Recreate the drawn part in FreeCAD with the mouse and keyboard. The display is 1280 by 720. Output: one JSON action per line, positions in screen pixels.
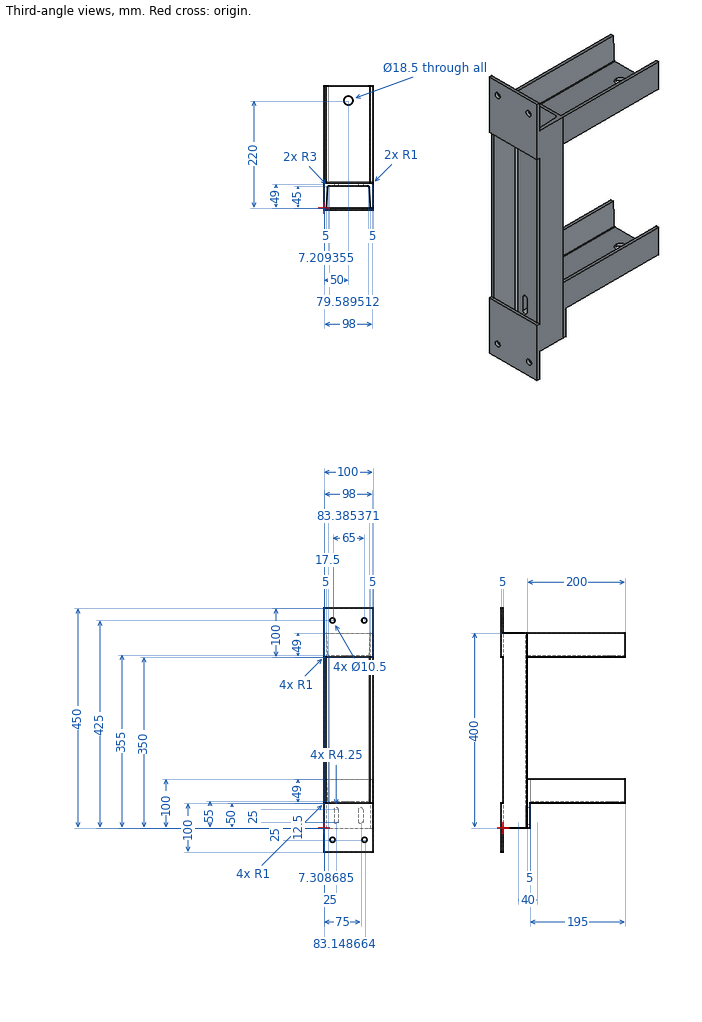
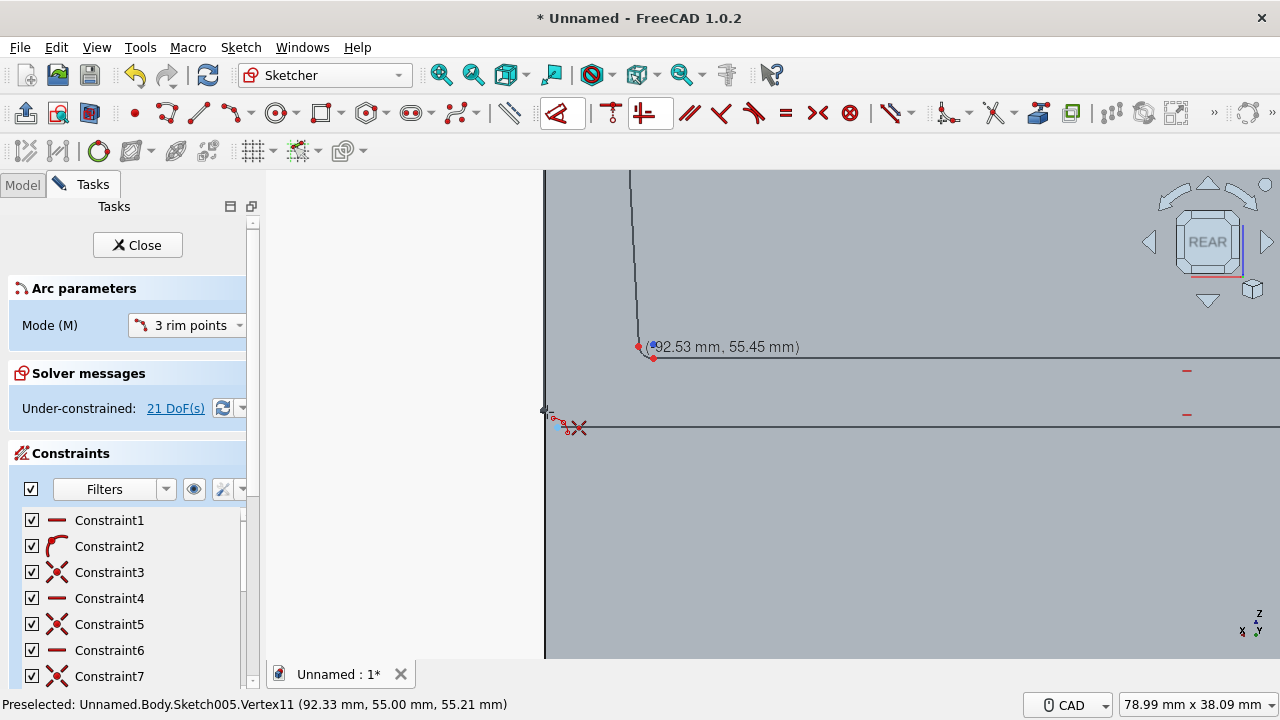
{"action": "left_click", "coordinate": [544, 410]}
{"action": "left_click", "coordinate": [558, 427]}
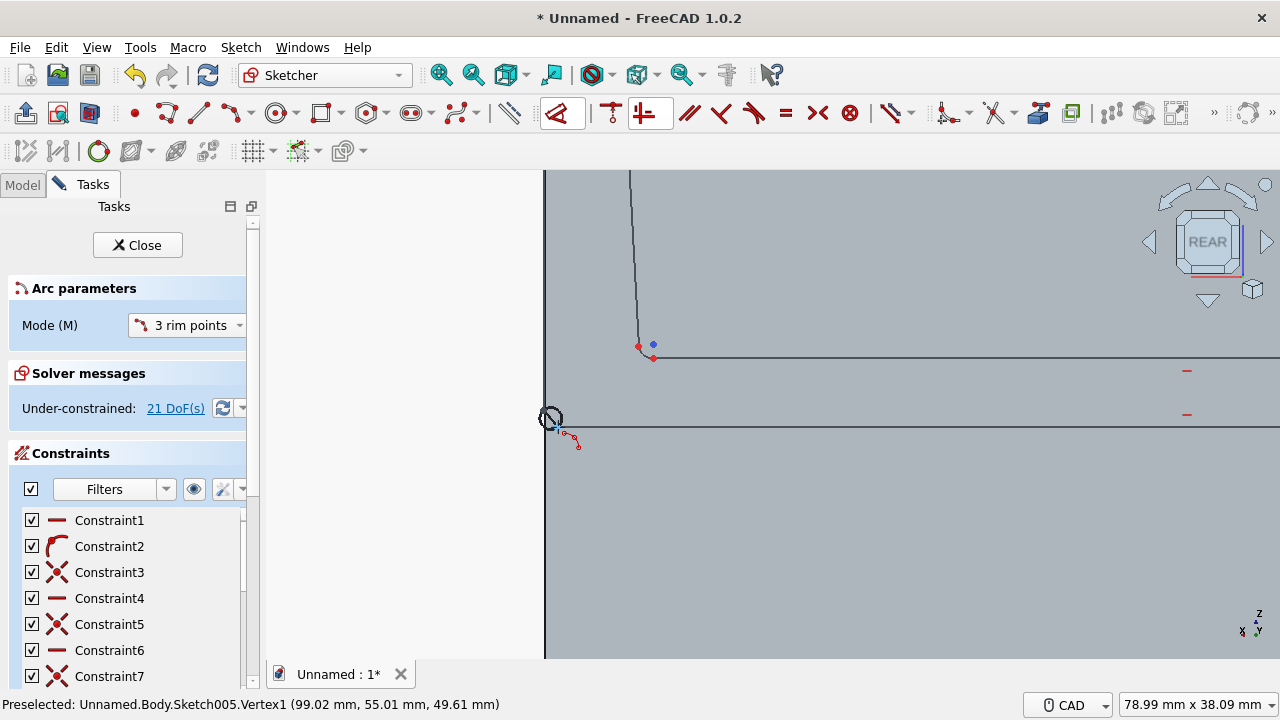
{"action": "scroll", "coordinate": [549, 418], "scroll_direction": "up", "scroll_amount": 8}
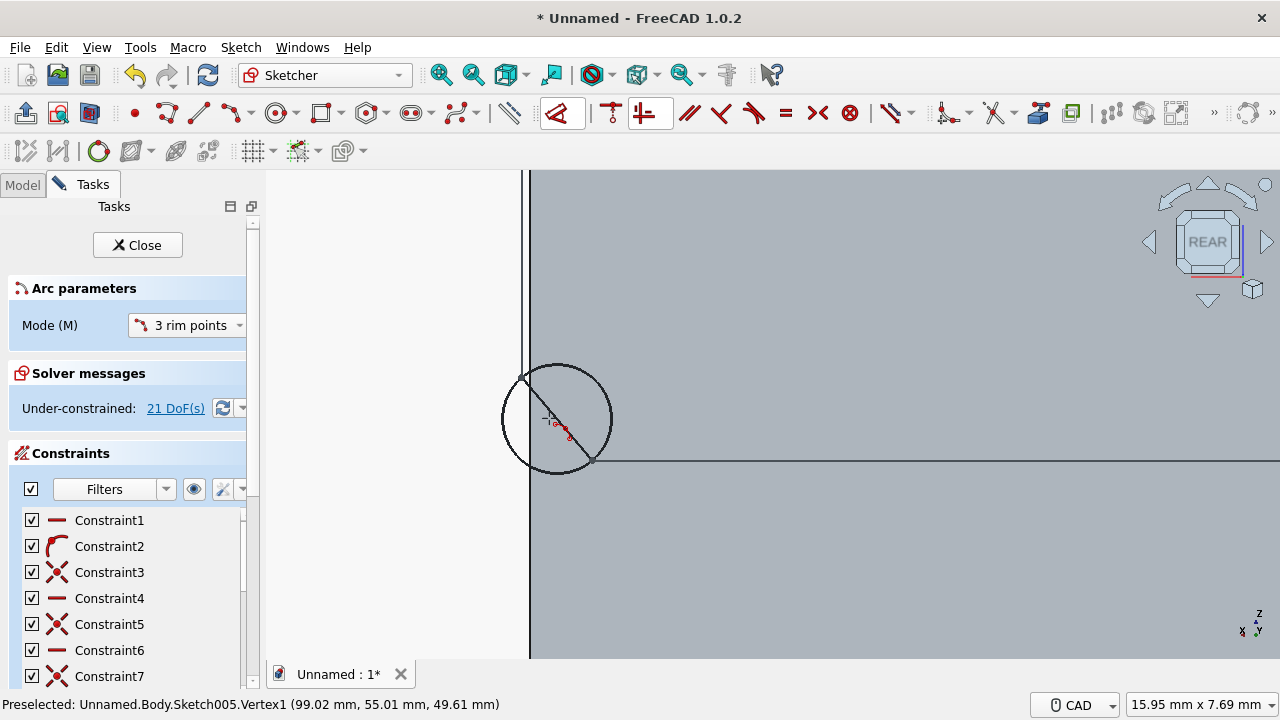
{"action": "left_click", "coordinate": [548, 417]}
{"action": "key", "text": "Escape"}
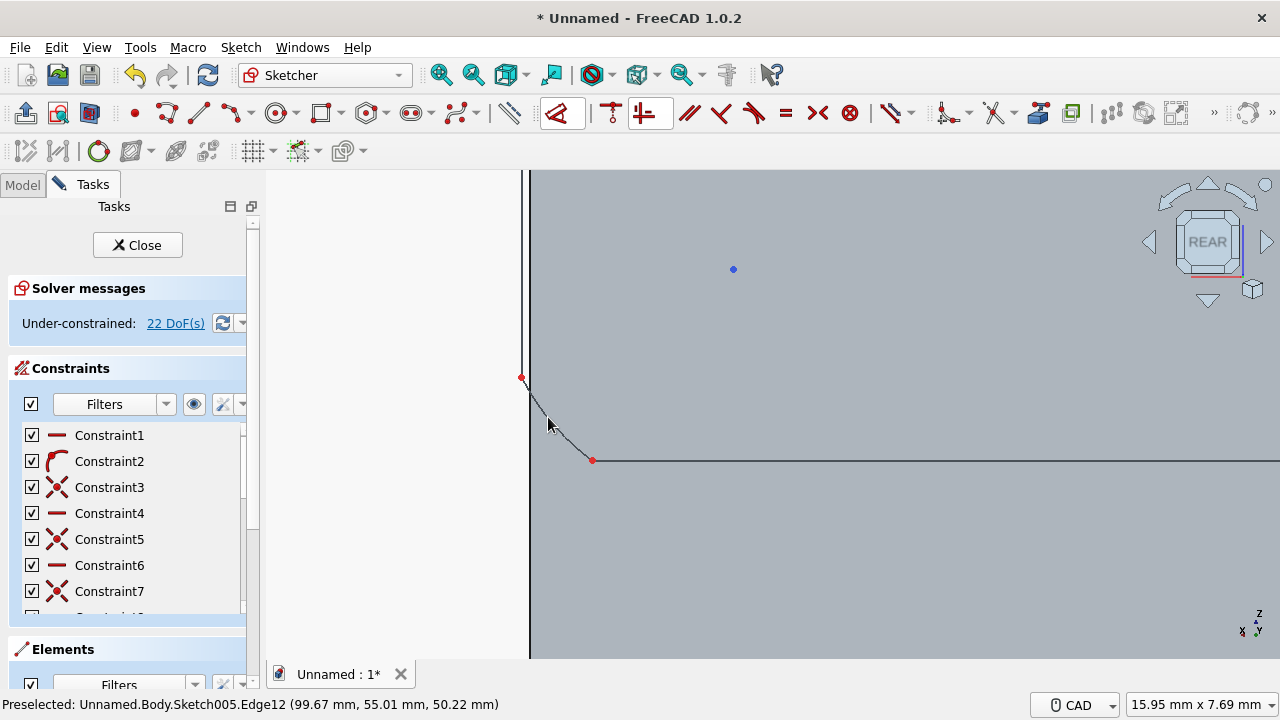
{"action": "scroll", "coordinate": [547, 413], "scroll_direction": "down", "scroll_amount": 15}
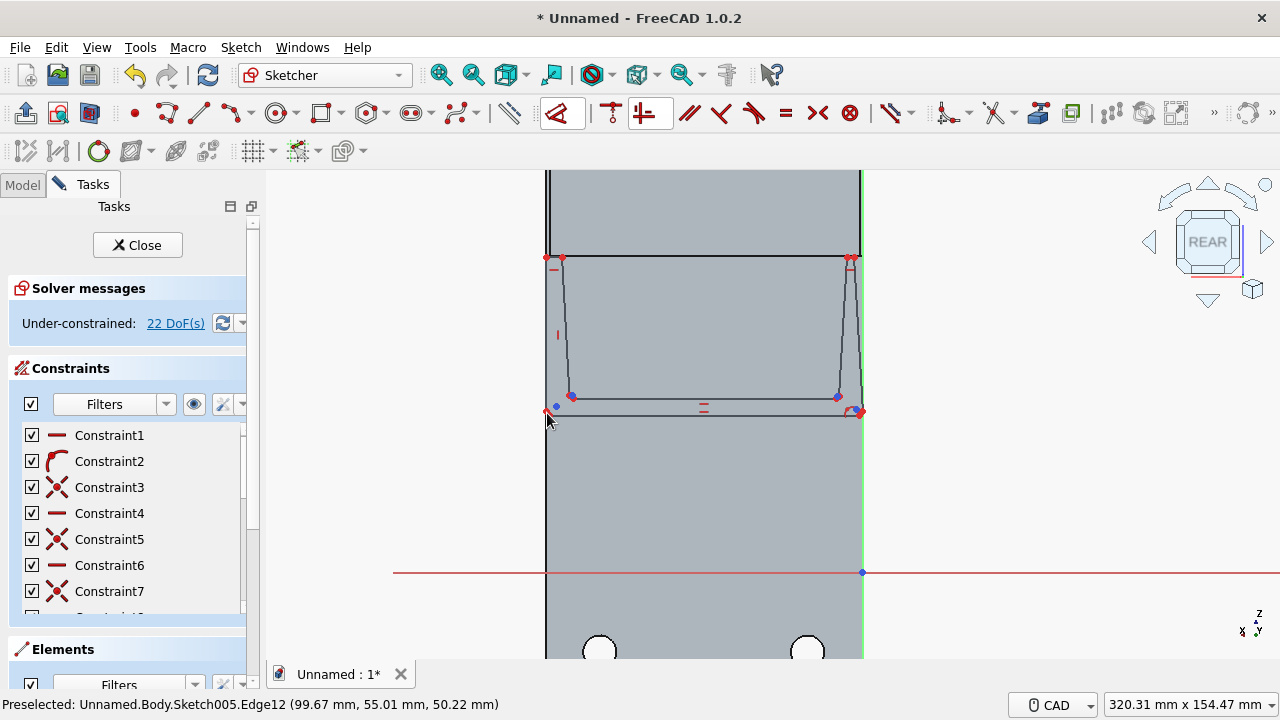
{"action": "left_click", "coordinate": [643, 416]}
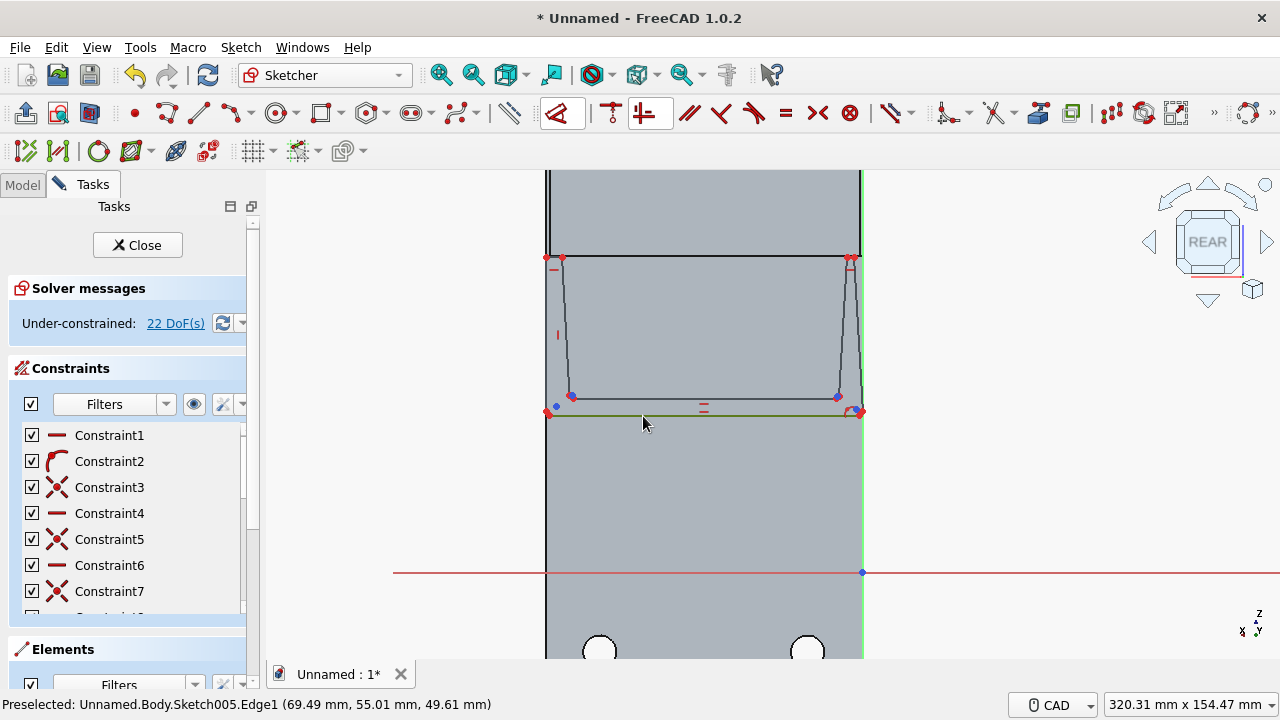
{"action": "scroll", "coordinate": [862, 414], "scroll_direction": "up", "scroll_amount": 9}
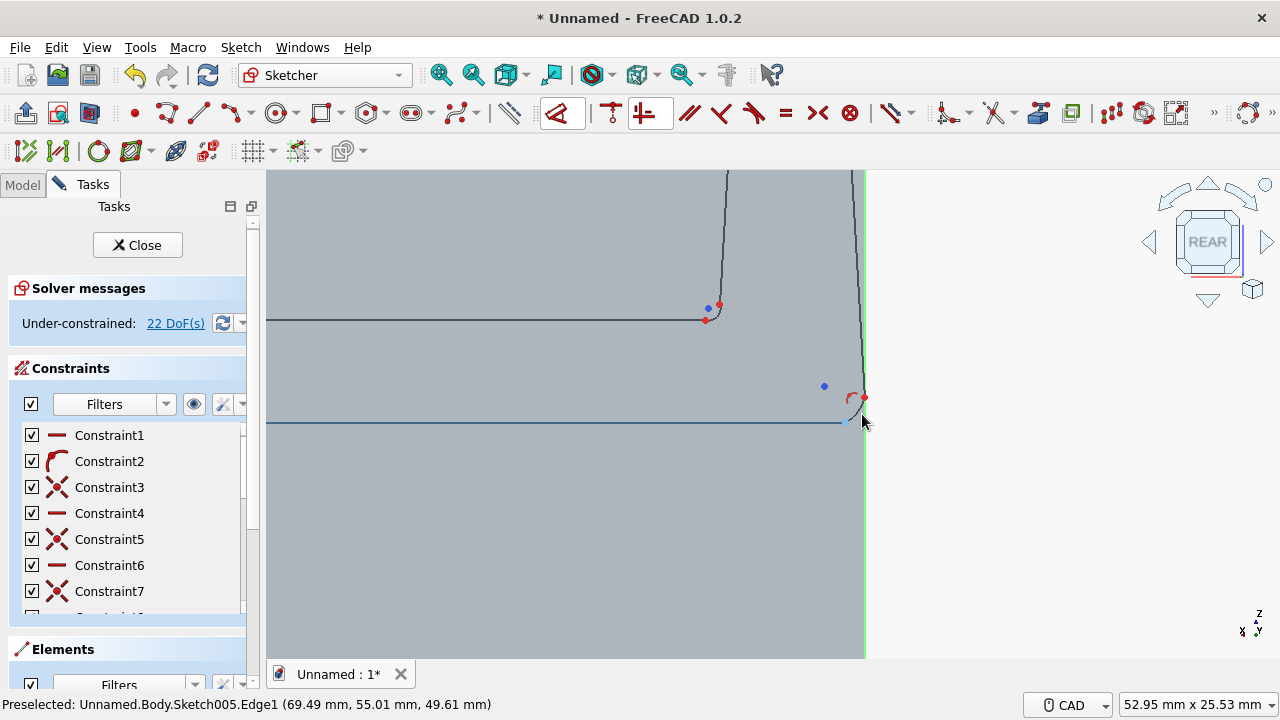
{"action": "left_click", "coordinate": [858, 412]}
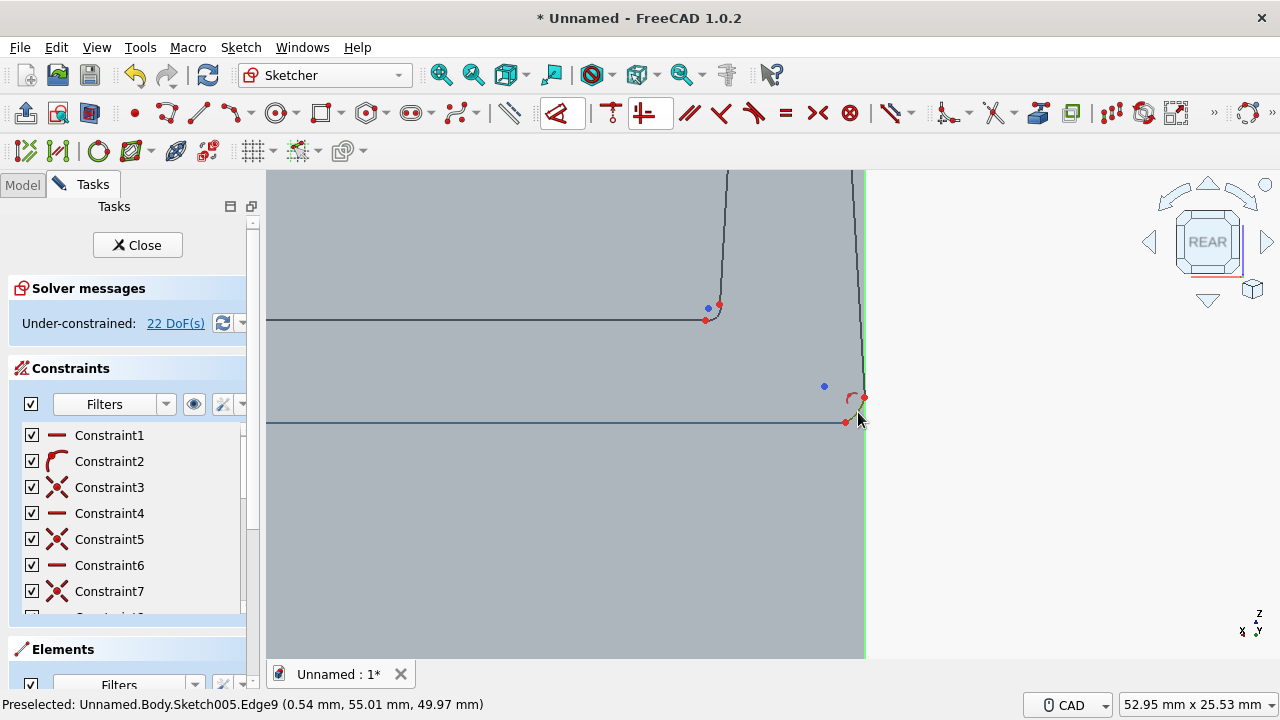
{"action": "key", "text": "t"}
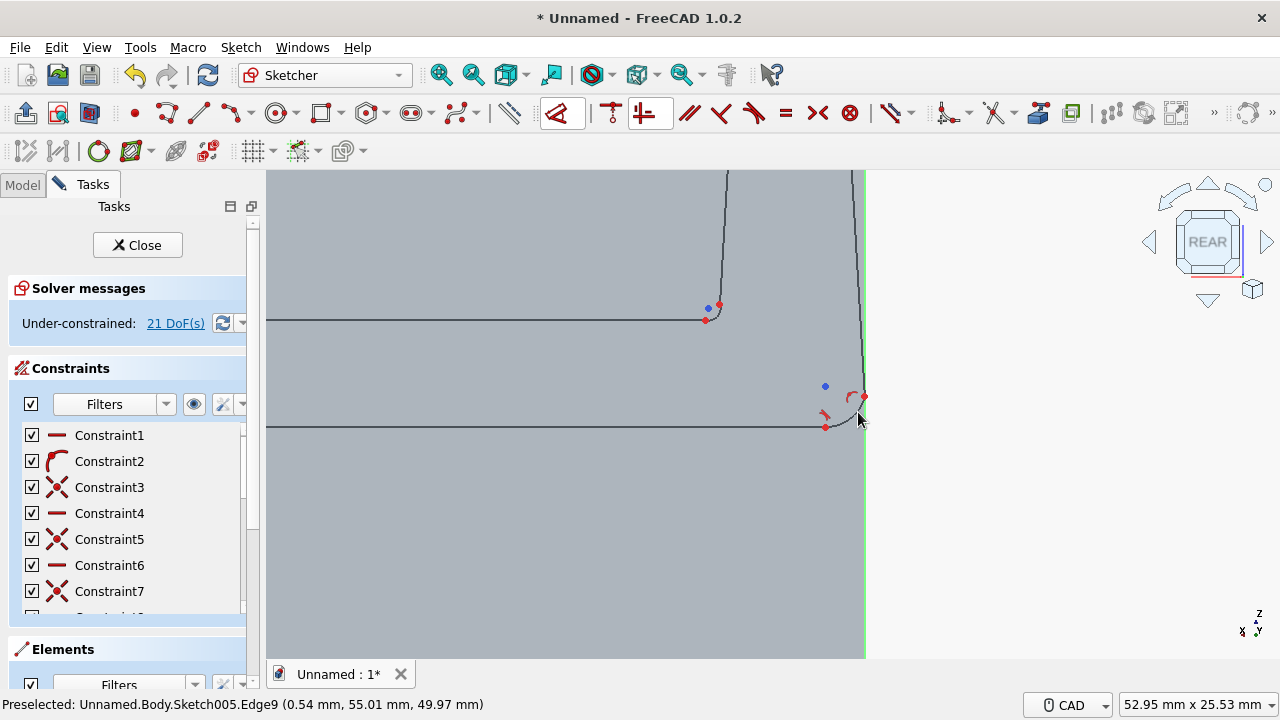
{"action": "scroll", "coordinate": [862, 414], "scroll_direction": "down", "scroll_amount": 9}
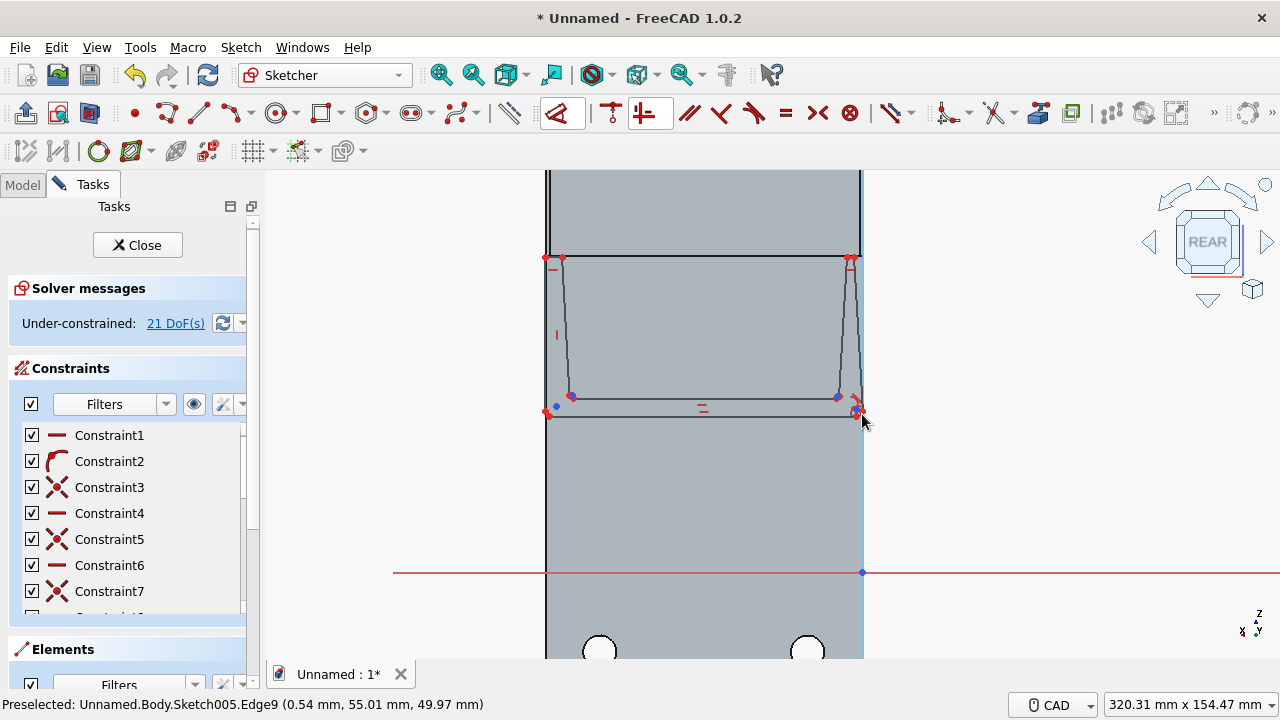
{"action": "left_click", "coordinate": [795, 417]}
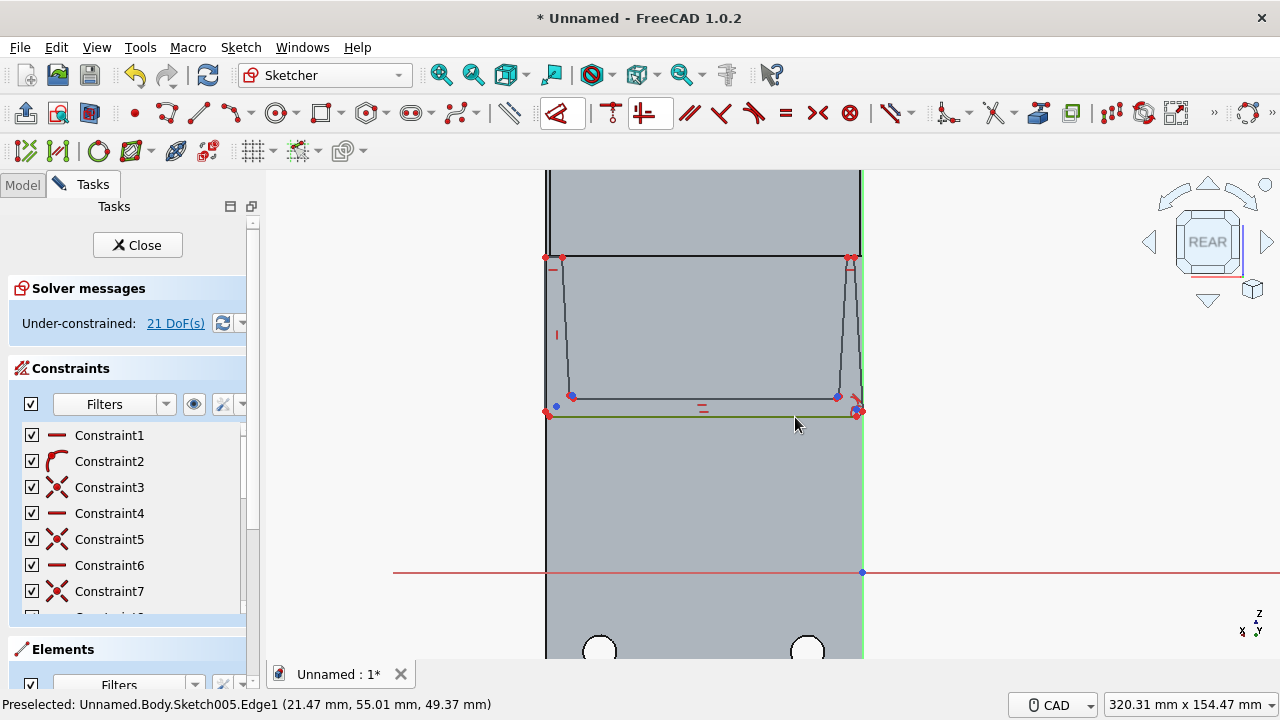
{"action": "scroll", "coordinate": [547, 414], "scroll_direction": "up", "scroll_amount": 8}